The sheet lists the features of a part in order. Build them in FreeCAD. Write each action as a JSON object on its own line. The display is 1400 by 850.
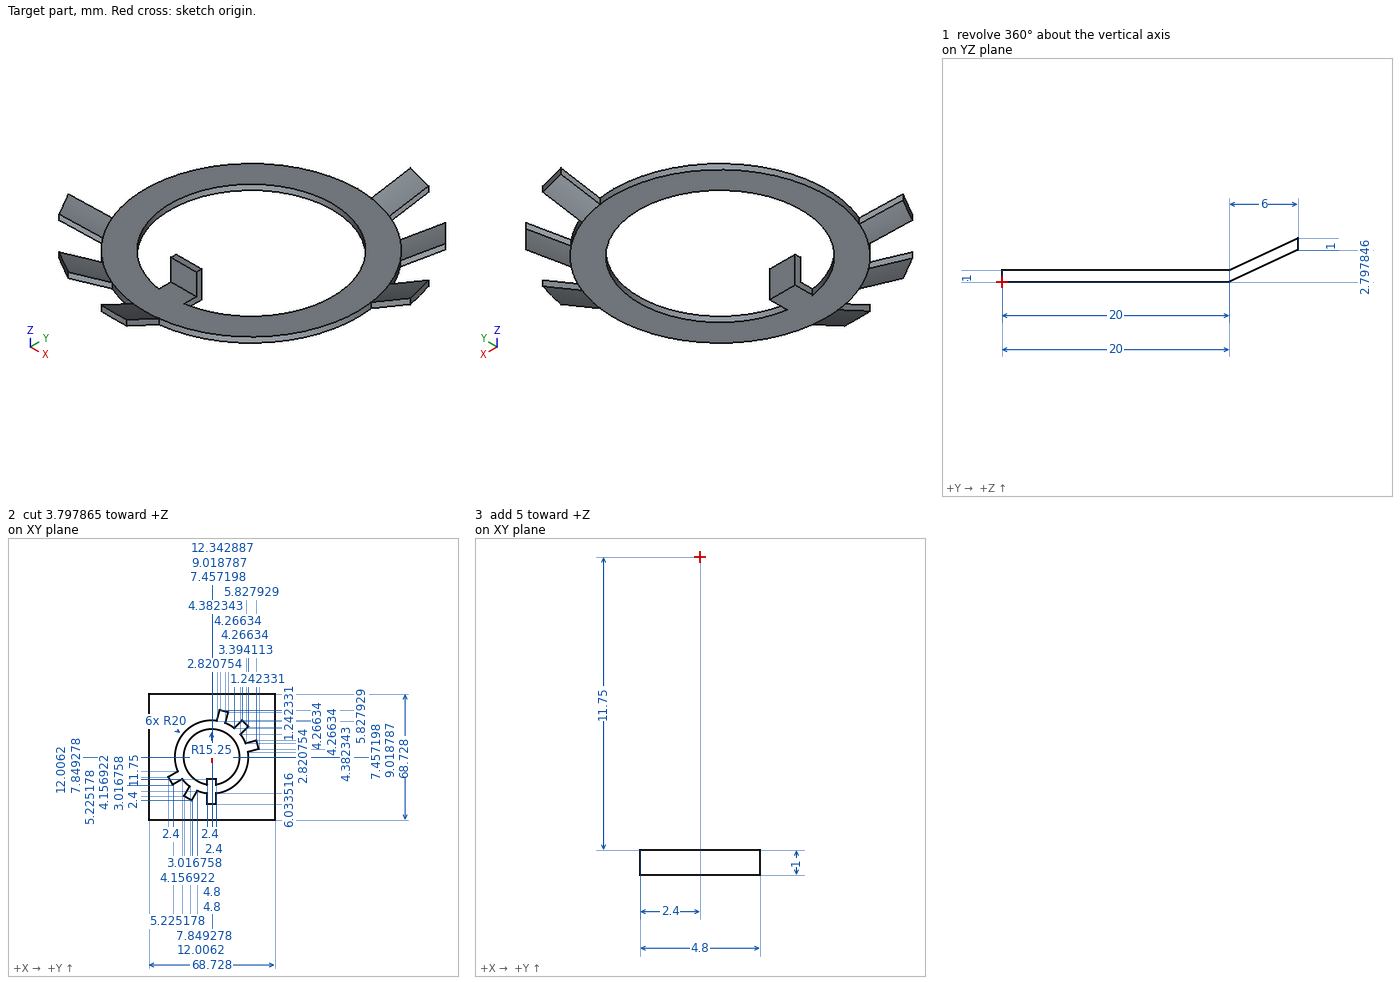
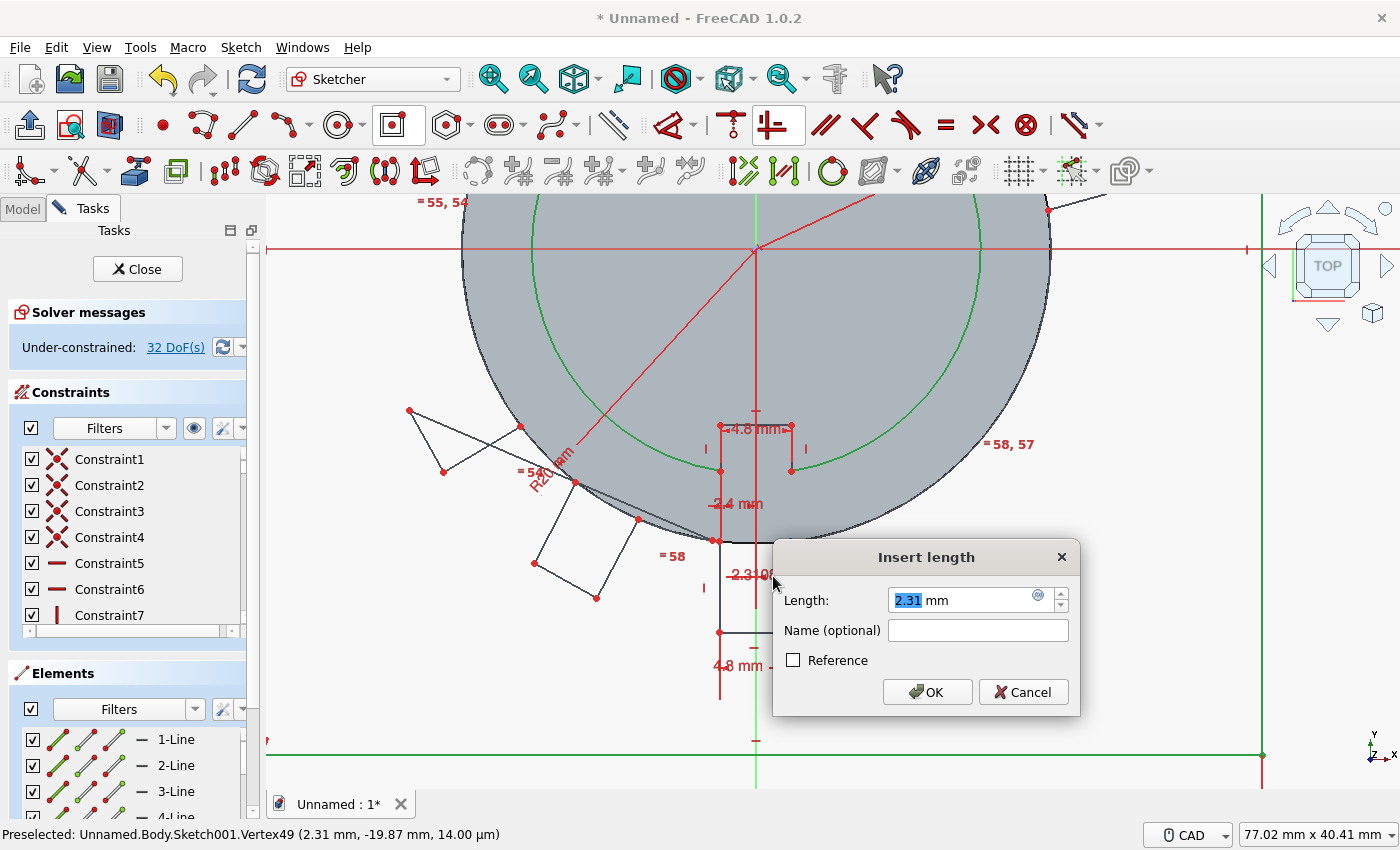
{"action": "type", "text": "2.4"}
{"action": "key", "text": "Return"}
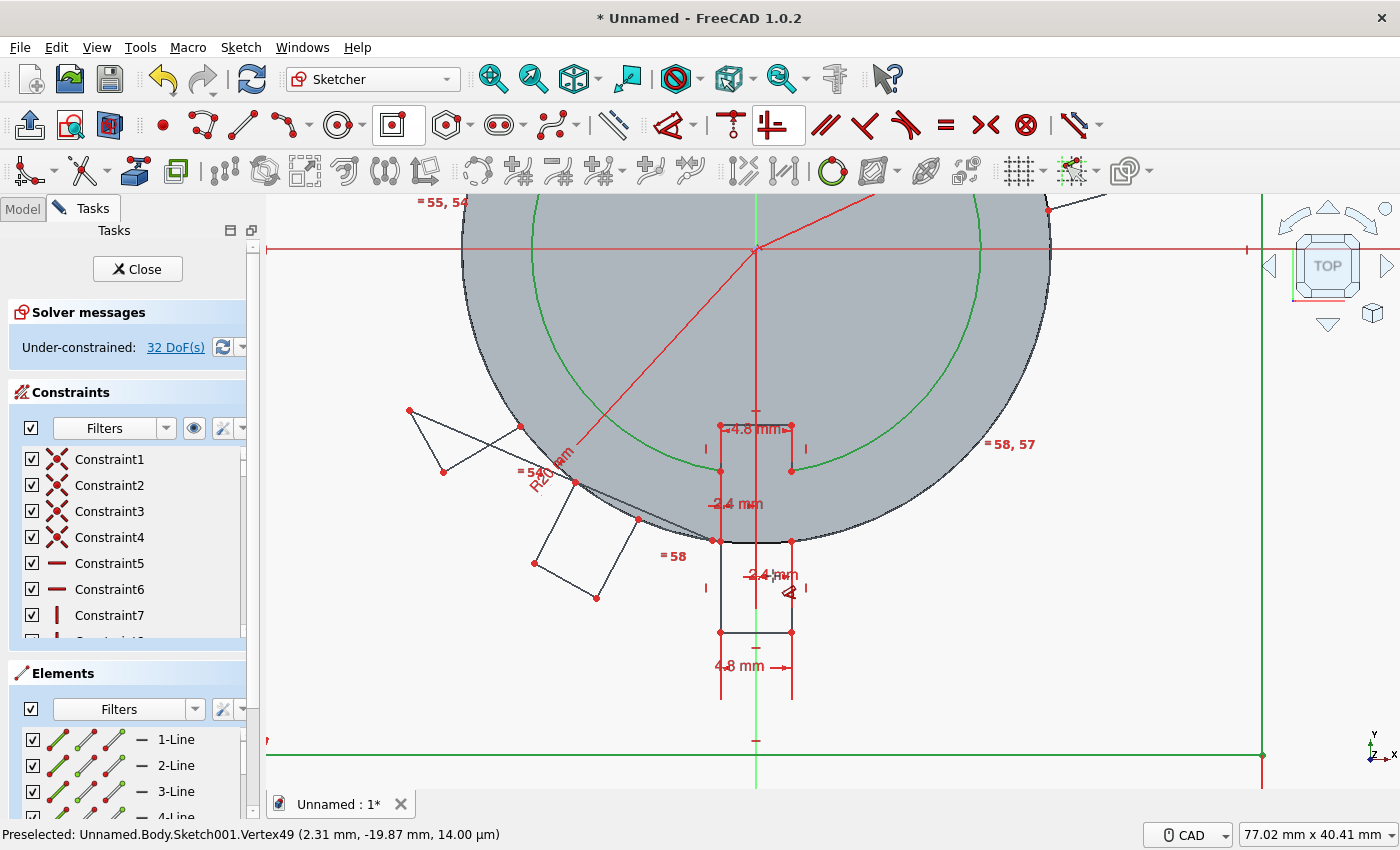
{"action": "left_click", "coordinate": [578, 588]}
{"action": "left_click", "coordinate": [501, 581]}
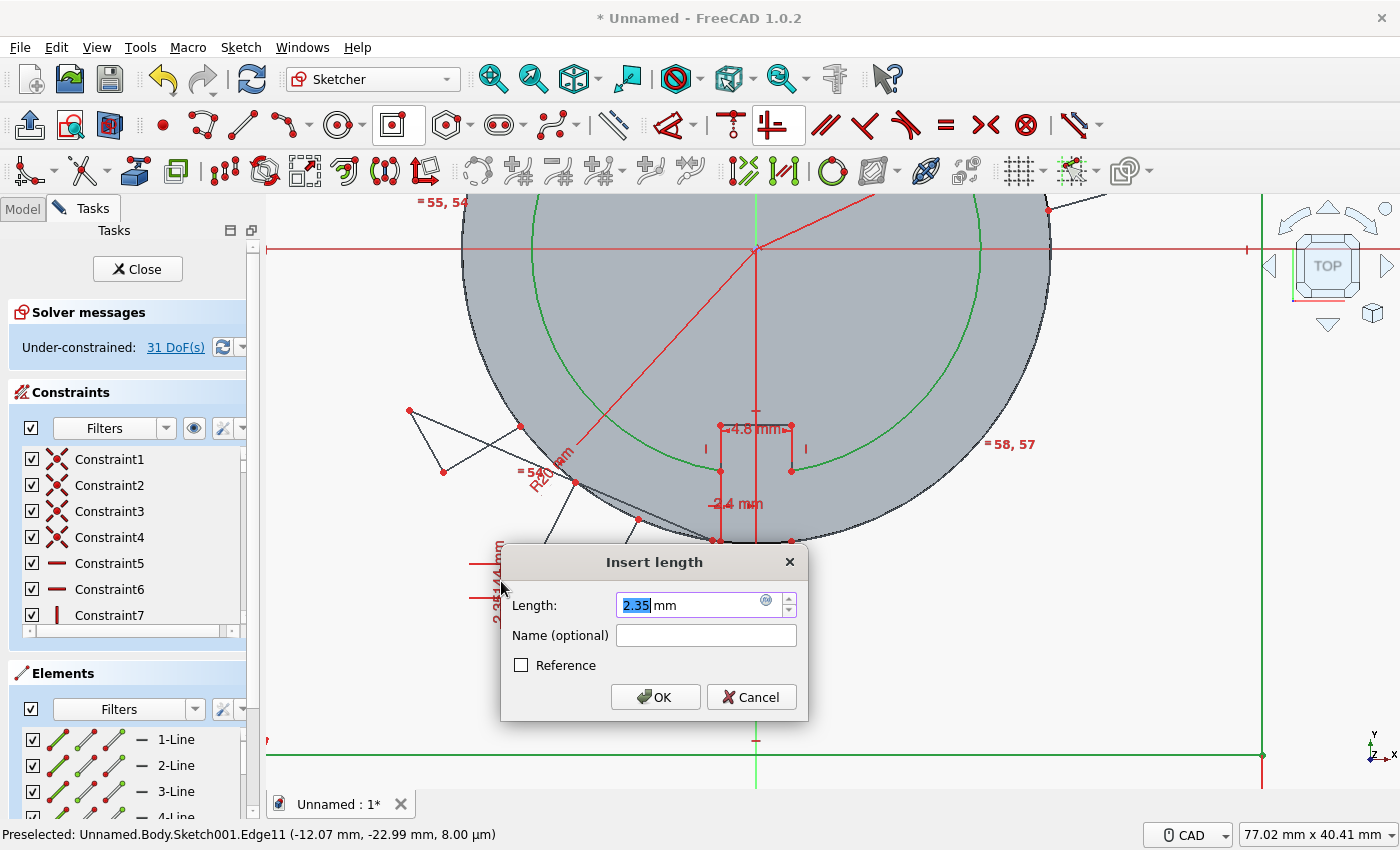
{"action": "type", "text": "2.4"}
{"action": "key", "text": "Return"}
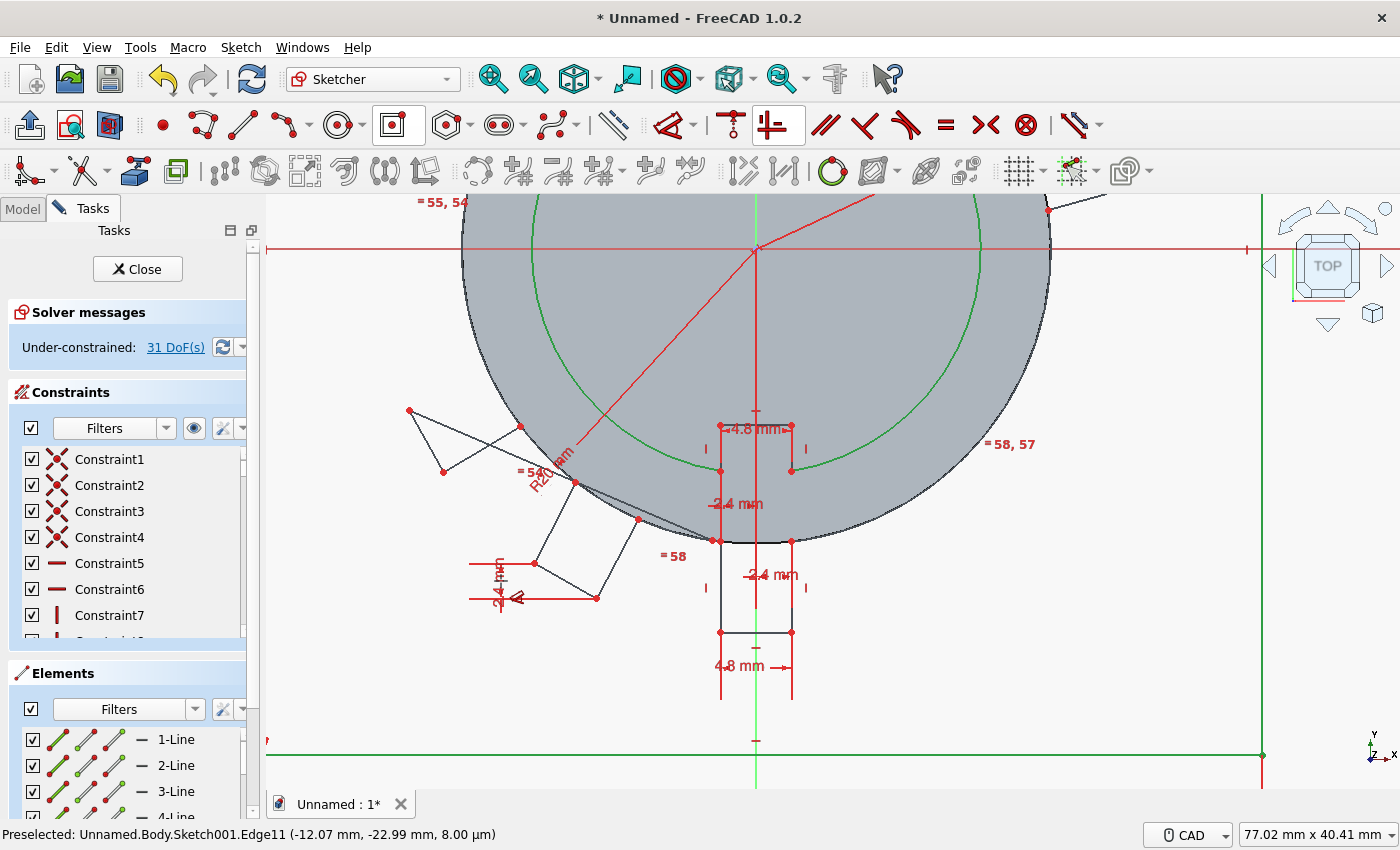
{"action": "left_click", "coordinate": [433, 454]}
{"action": "left_click", "coordinate": [426, 506]}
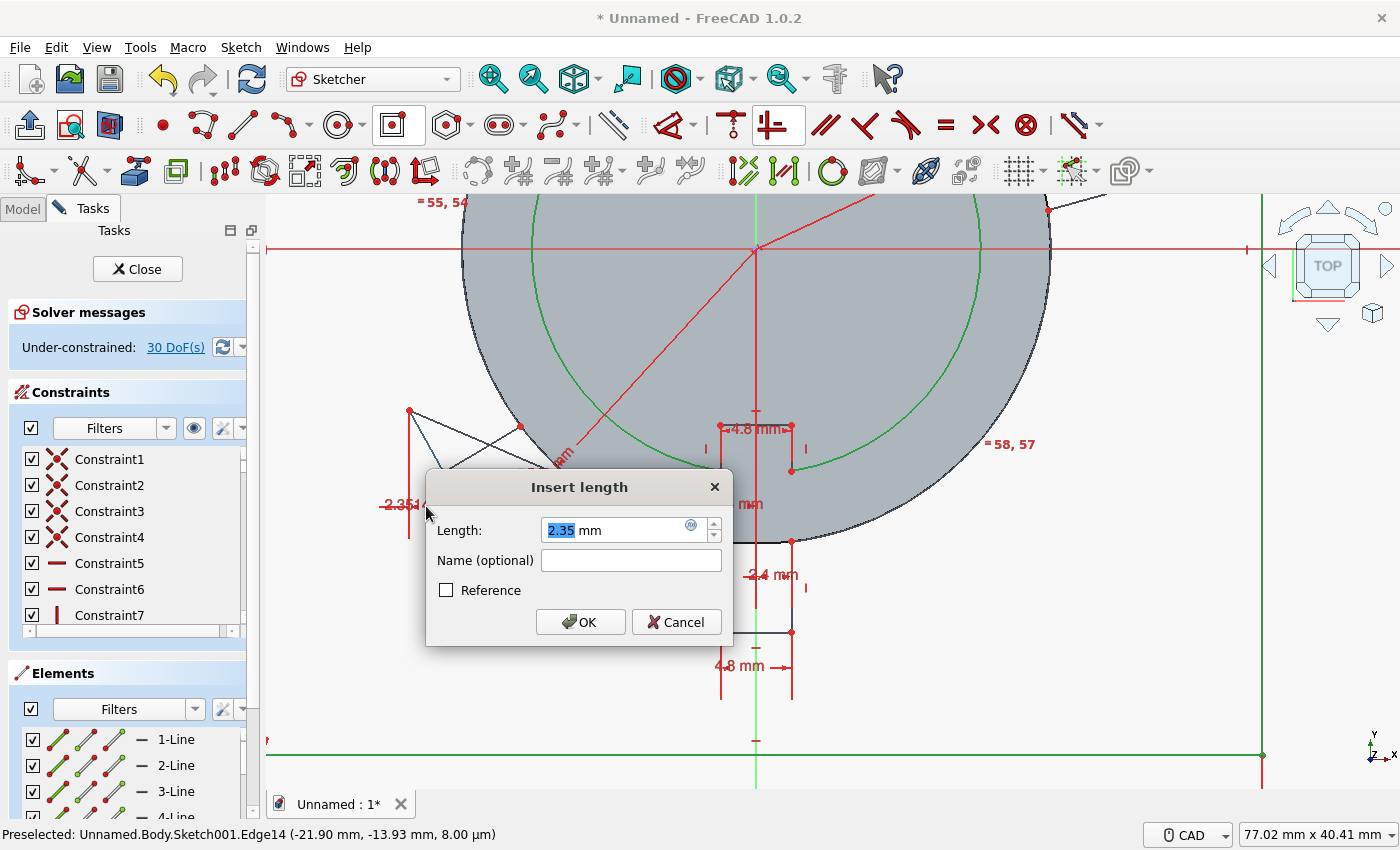
{"action": "type", "text": "2.4"}
{"action": "key", "text": "Return"}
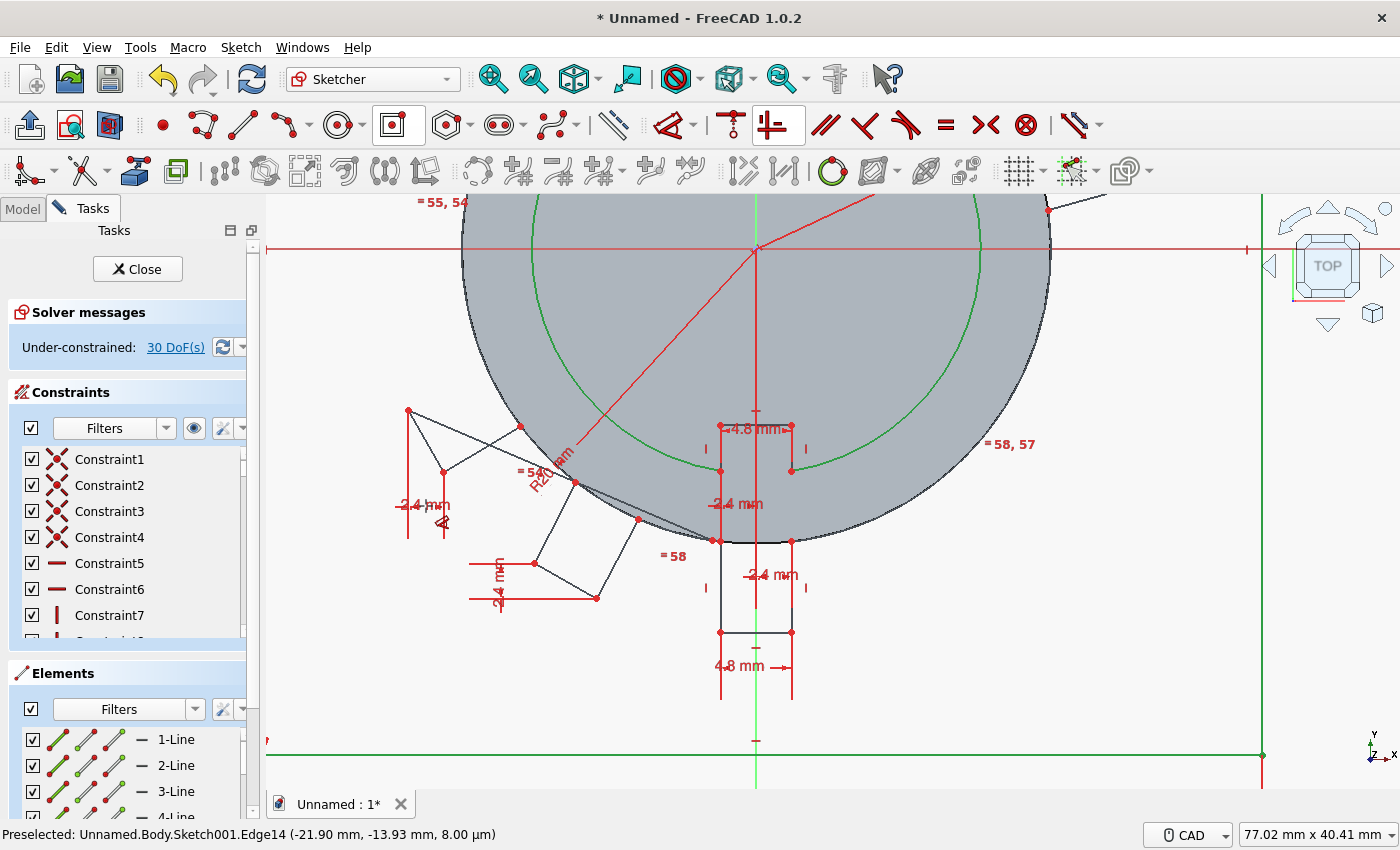
{"action": "left_click", "coordinate": [721, 425]}
{"action": "left_click", "coordinate": [687, 337]}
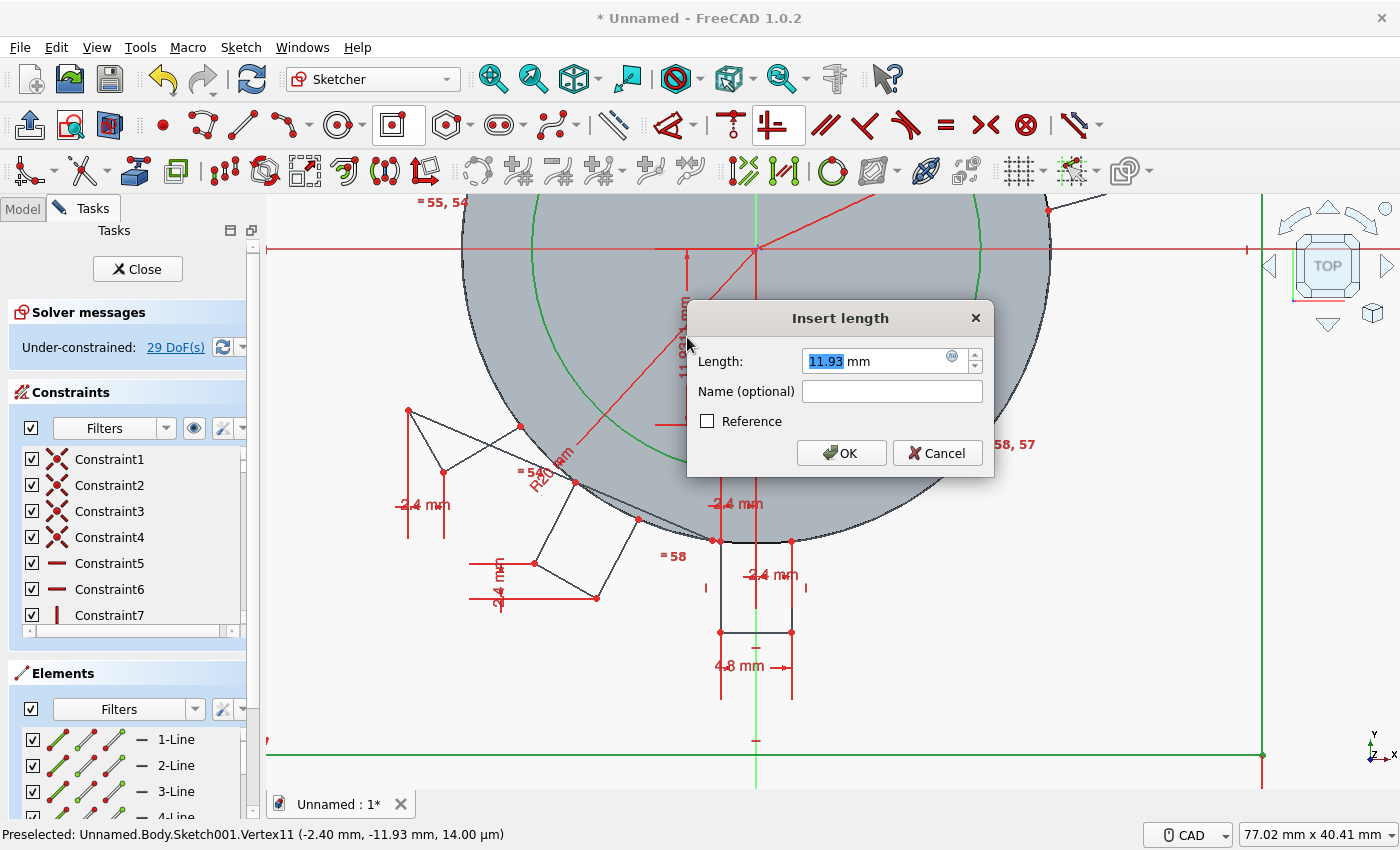
{"action": "type", "text": "11.75"}
{"action": "key", "text": "Return"}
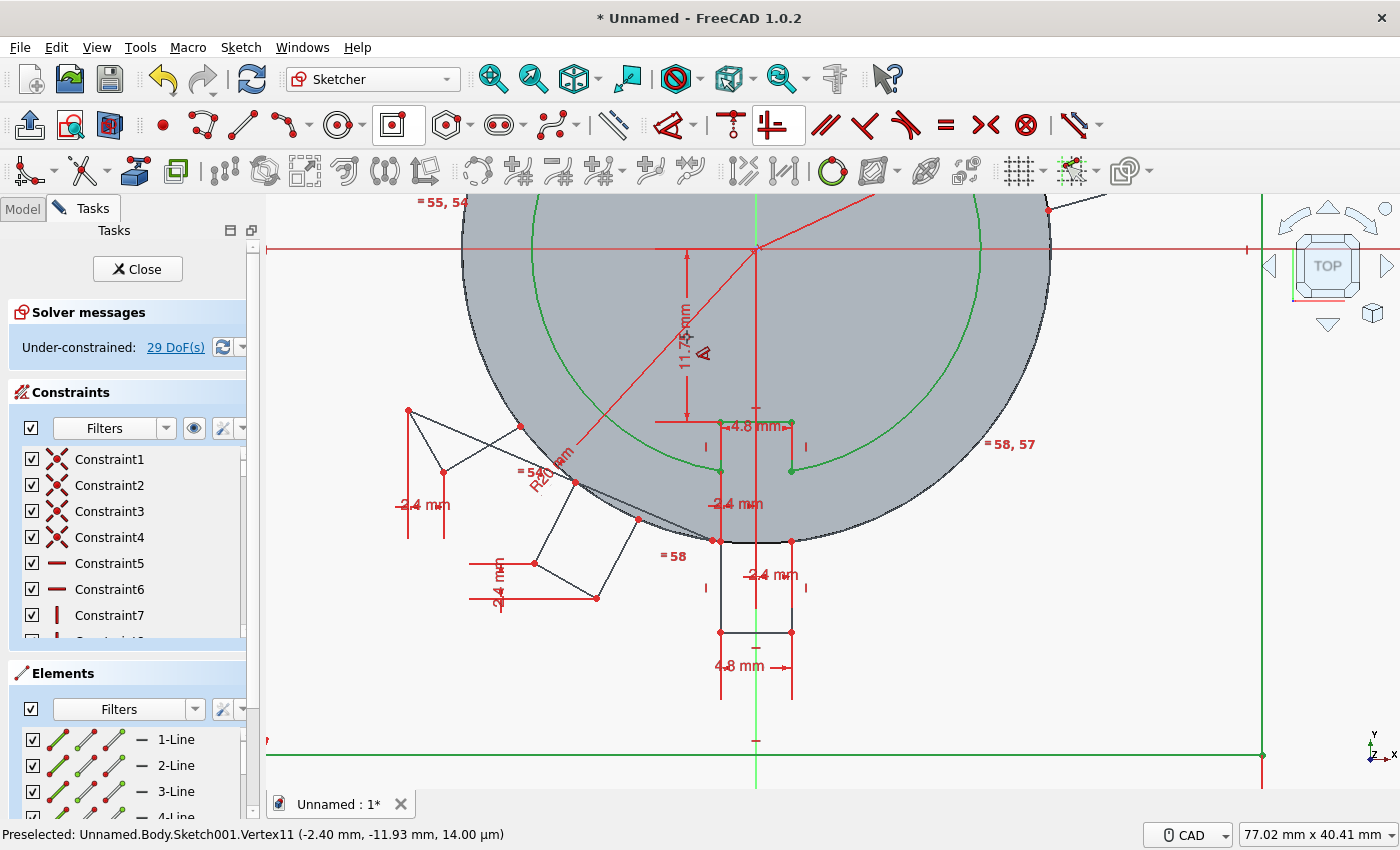
{"action": "left_click", "coordinate": [792, 569]}
{"action": "left_click", "coordinate": [826, 608]}